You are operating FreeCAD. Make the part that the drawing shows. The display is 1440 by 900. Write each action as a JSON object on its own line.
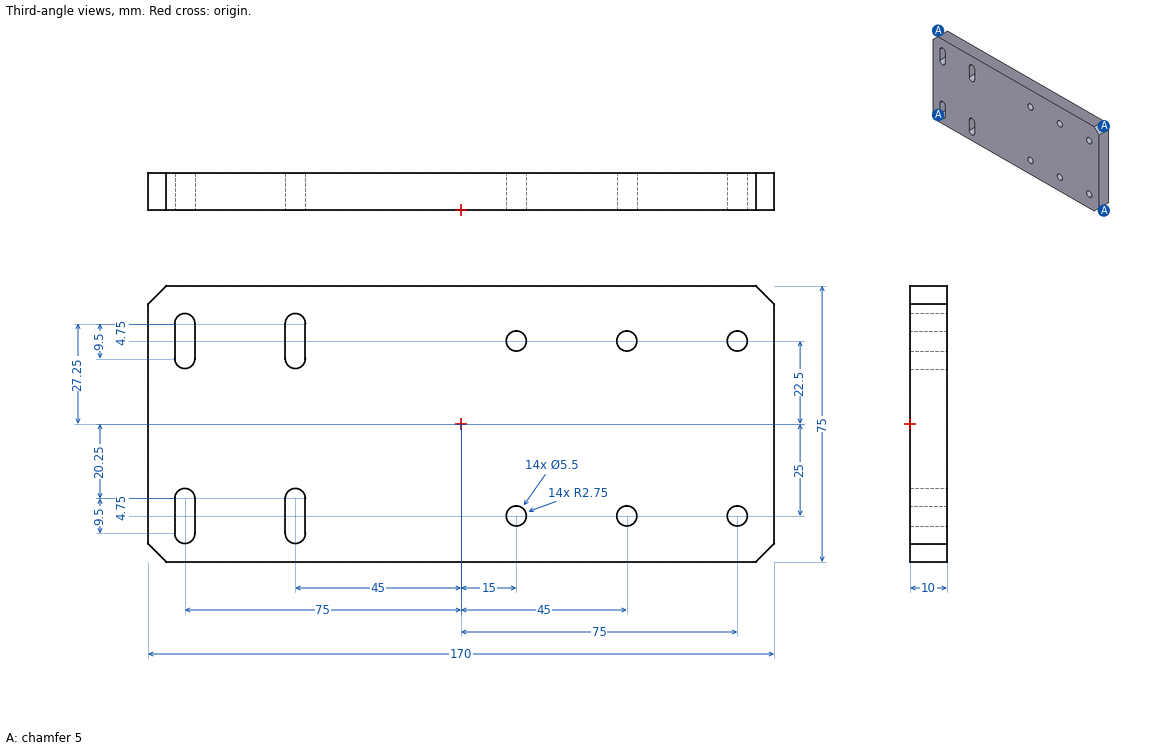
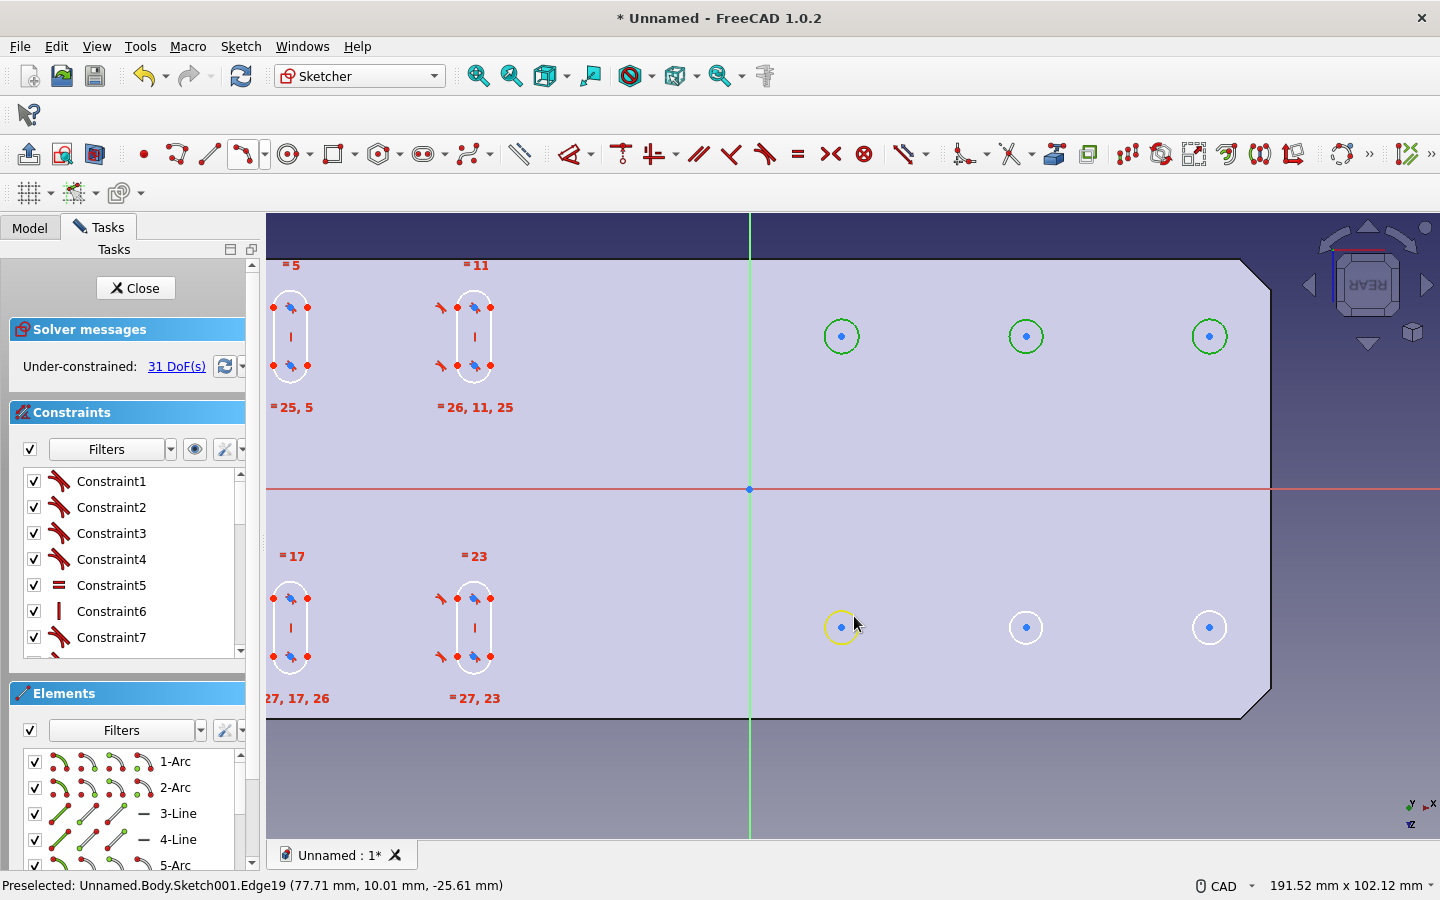
{"action": "left_click", "coordinate": [853, 616]}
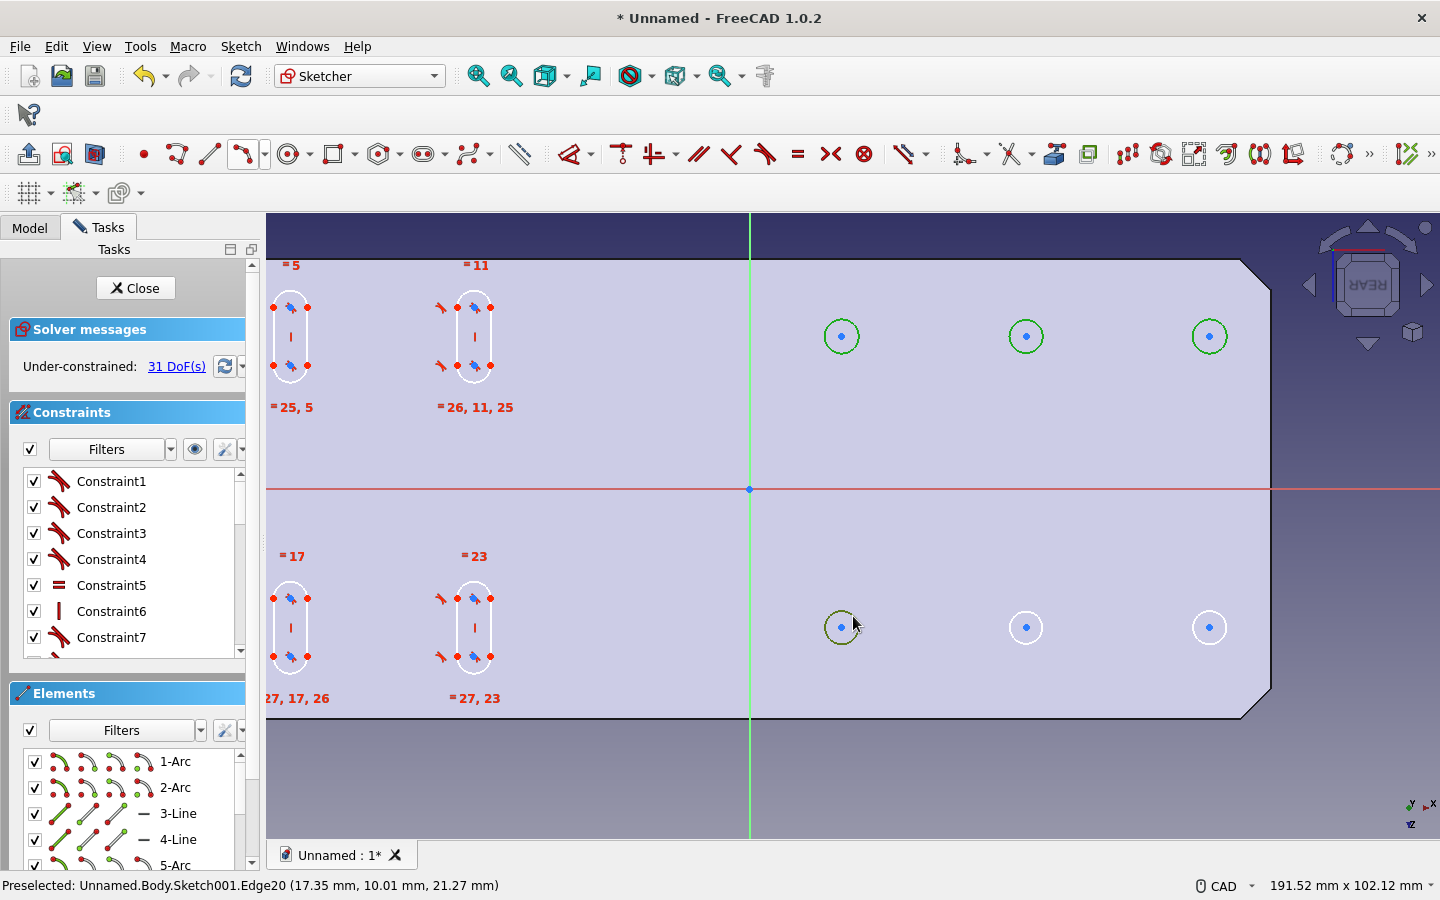
{"action": "left_click", "coordinate": [1037, 616]}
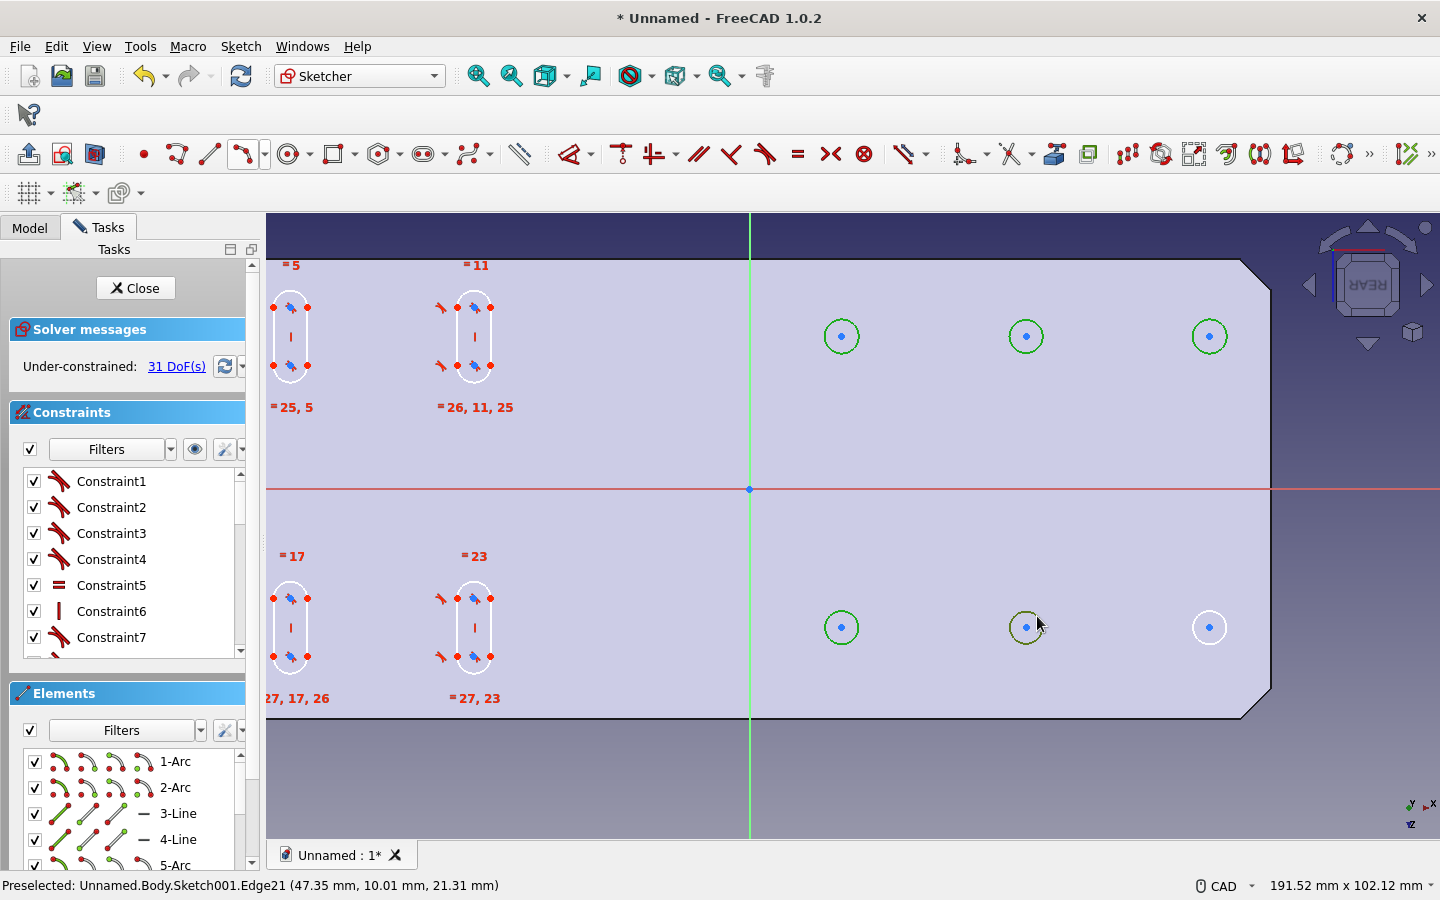
{"action": "left_click", "coordinate": [1221, 616]}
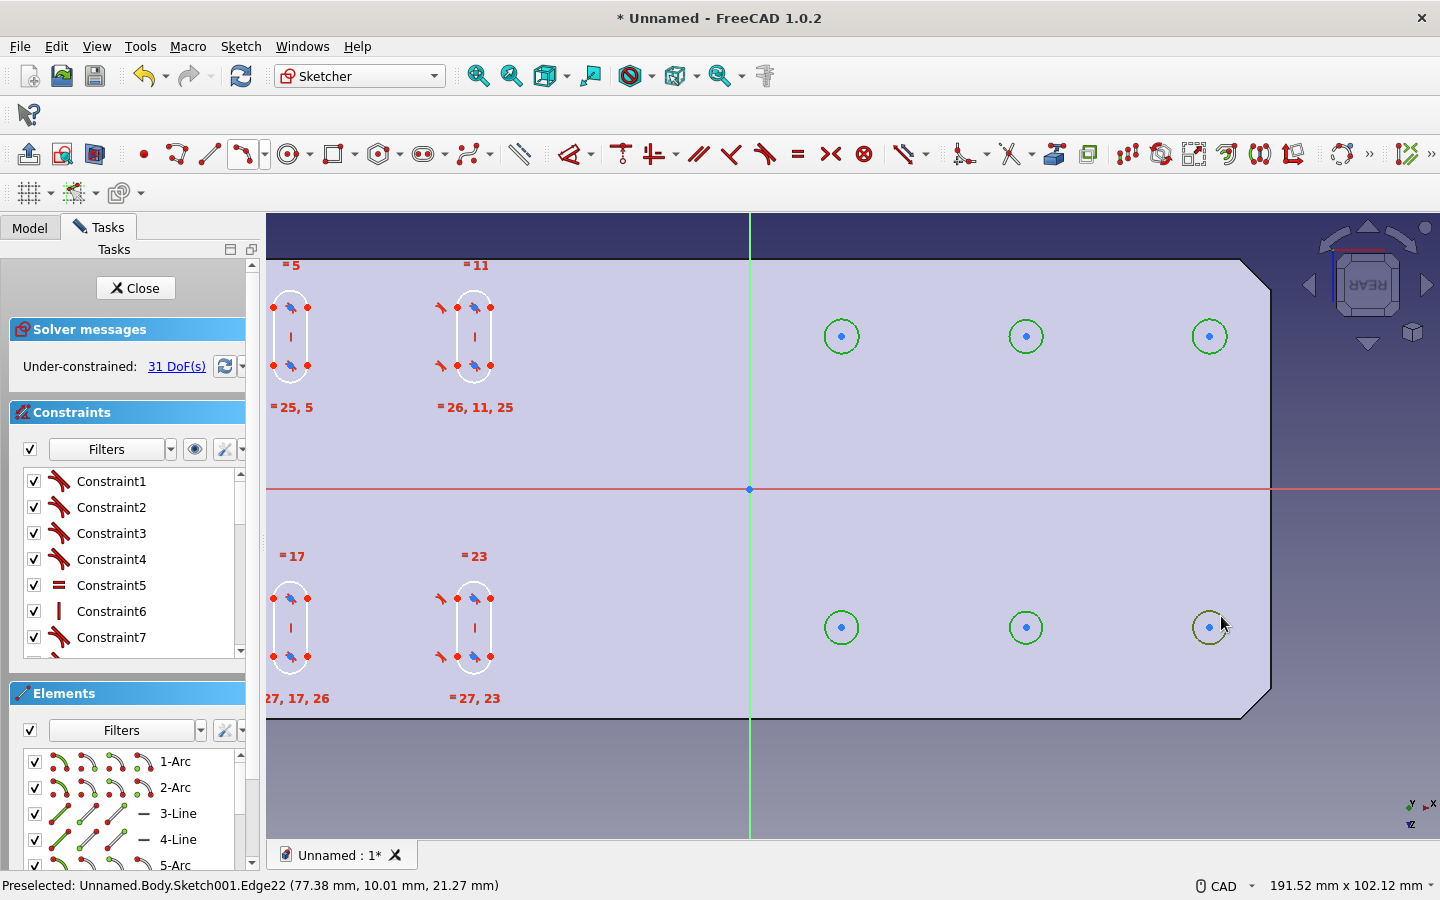
{"action": "left_click", "coordinate": [798, 154]}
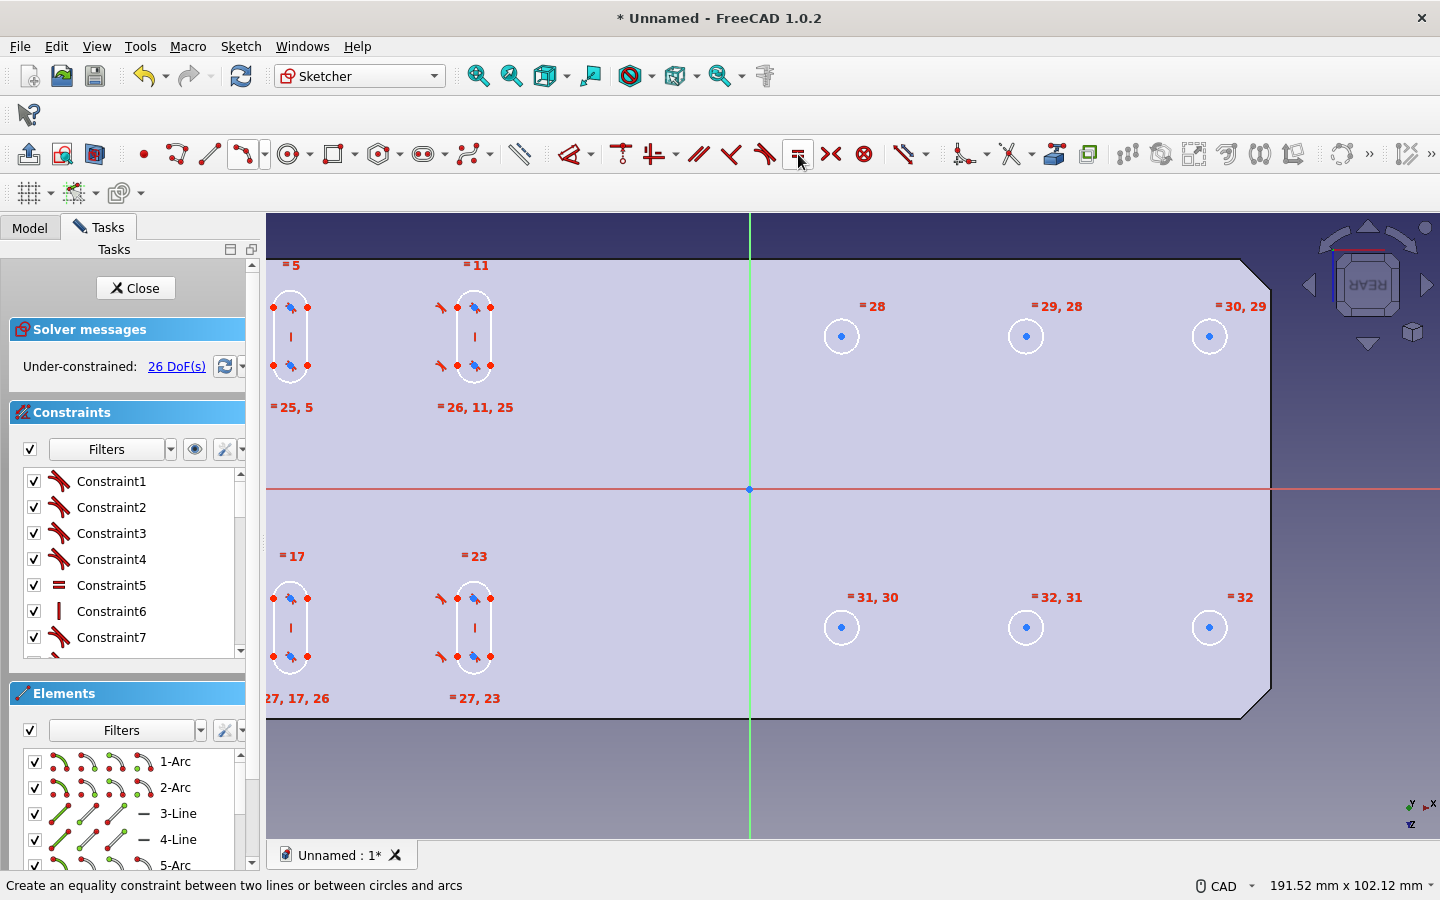
{"action": "key", "text": "d"}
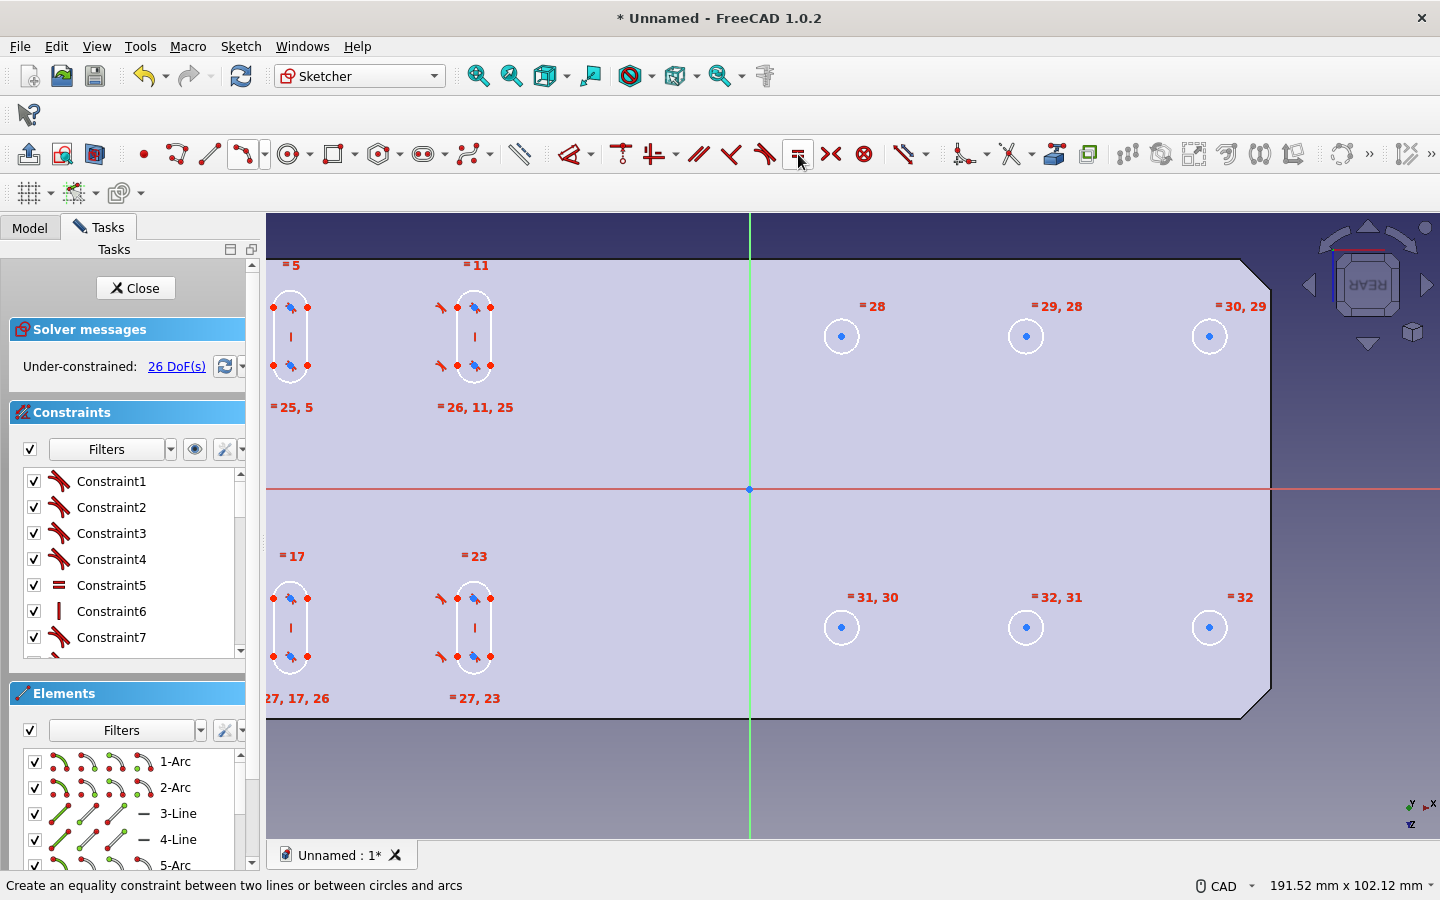
{"action": "scroll", "coordinate": [300, 379], "scroll_direction": "up", "scroll_amount": 5}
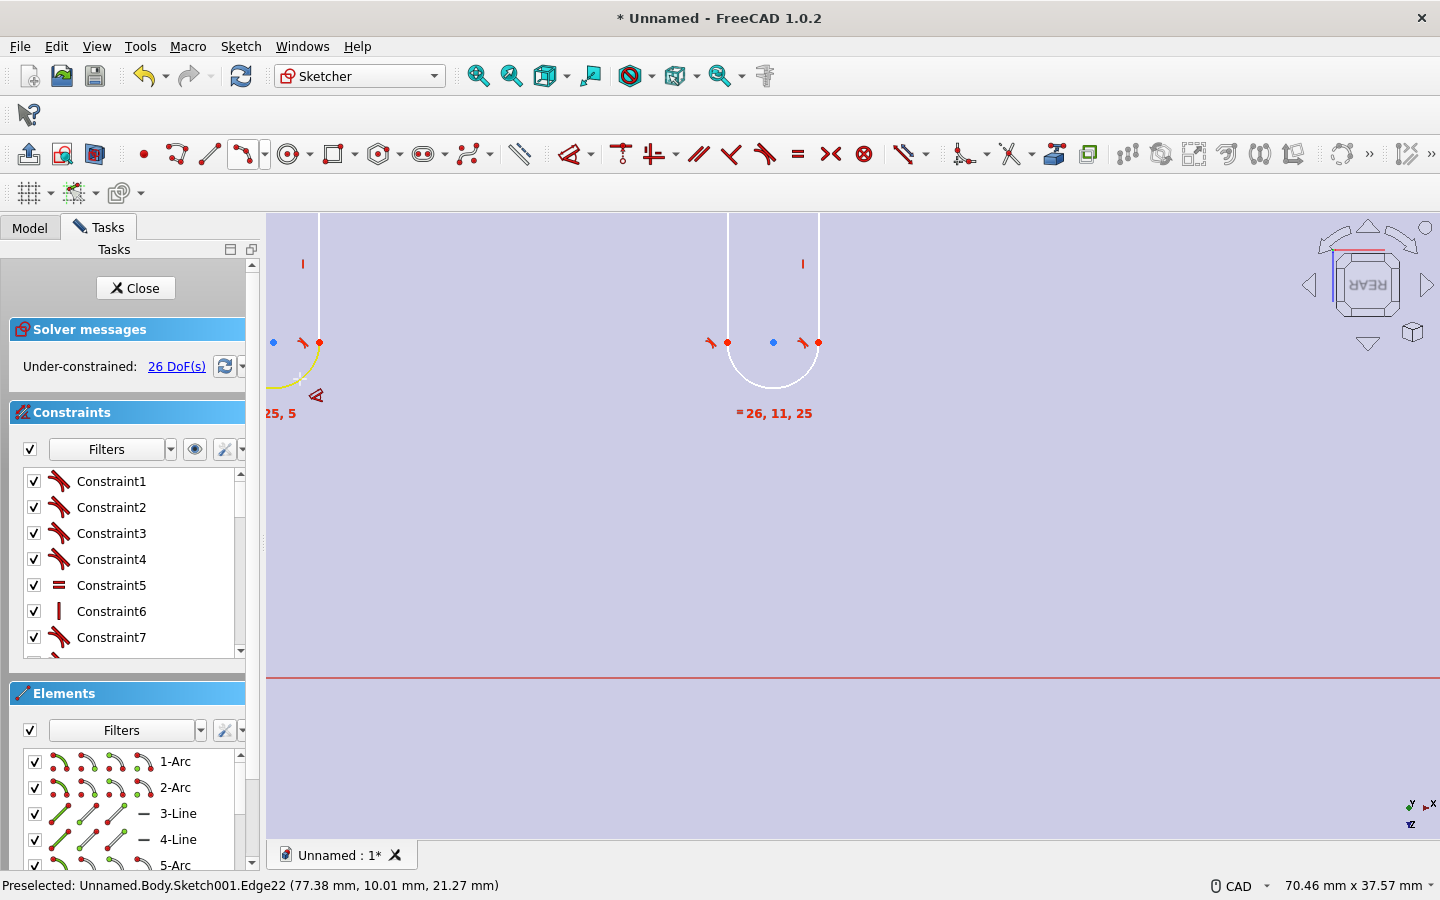
{"action": "left_click", "coordinate": [301, 380]}
{"action": "left_click", "coordinate": [320, 406]}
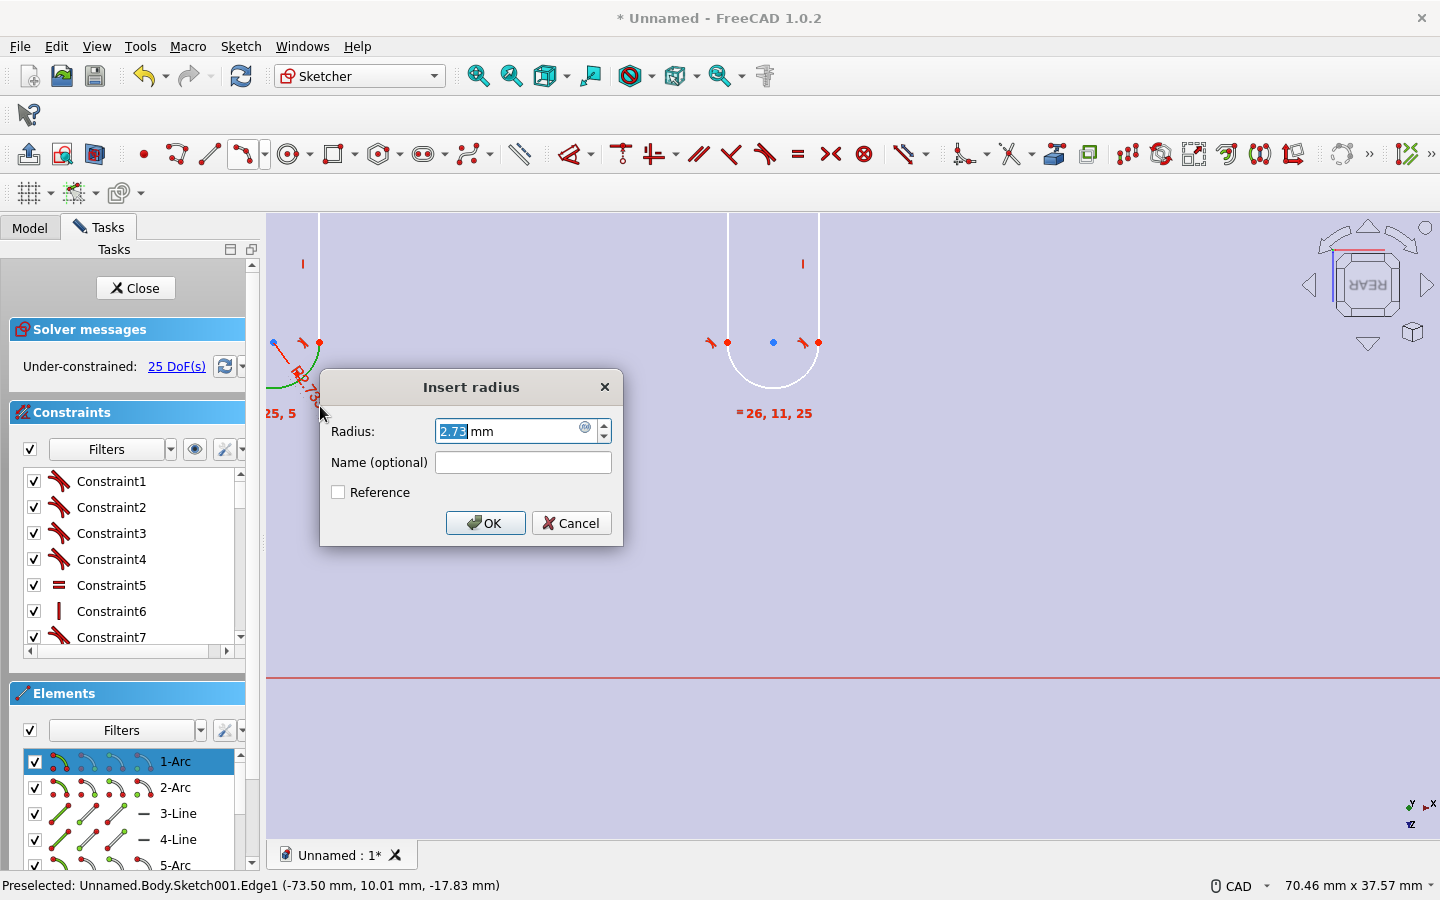
{"action": "type", "text": "2.75"}
{"action": "key", "text": "Return"}